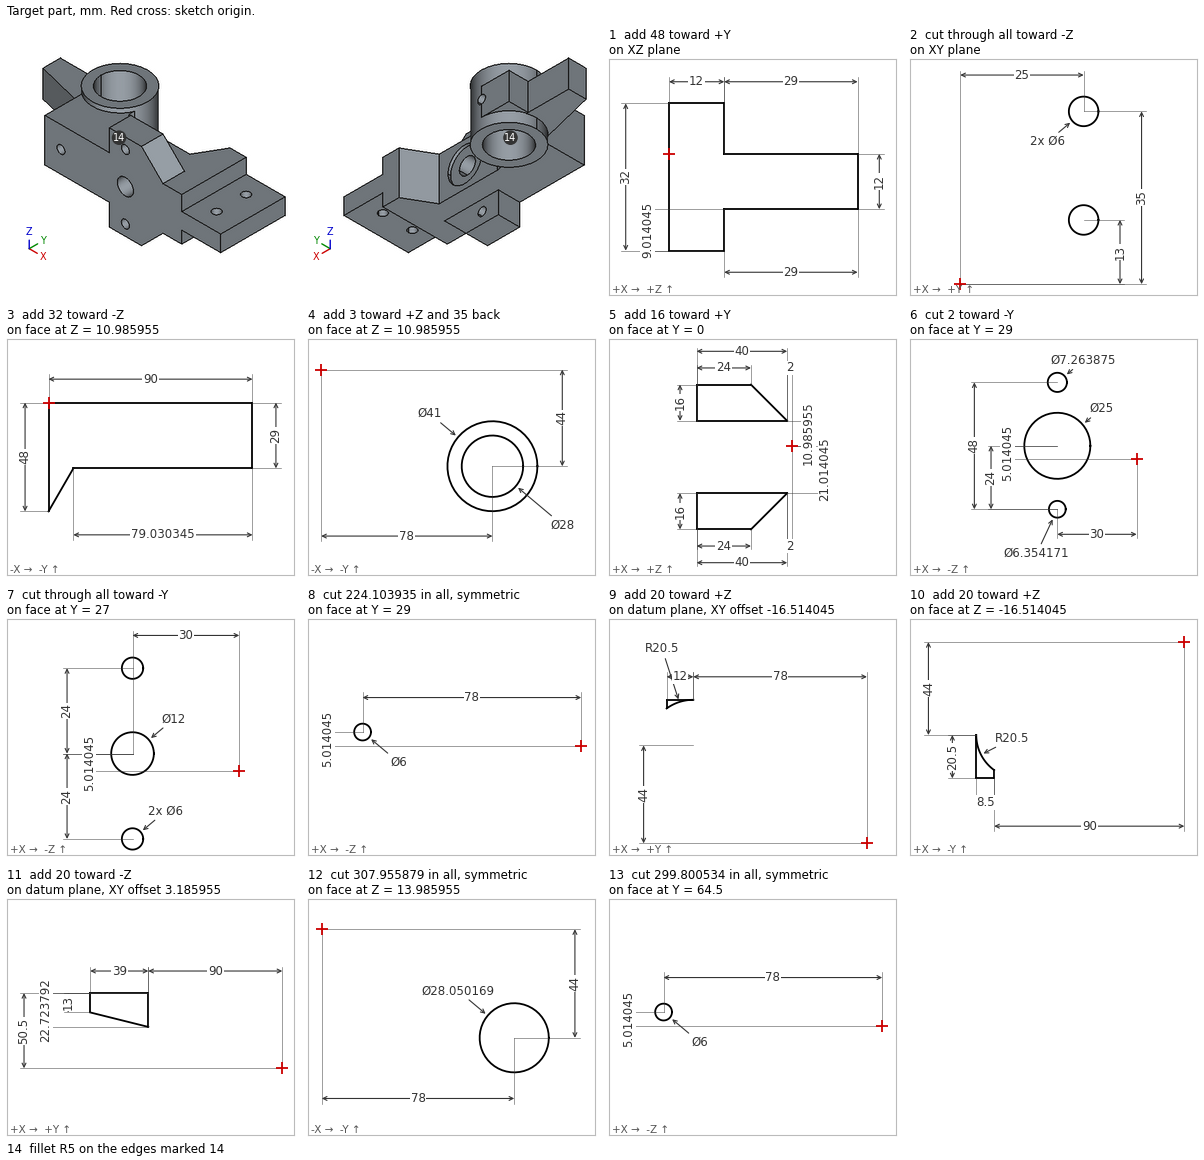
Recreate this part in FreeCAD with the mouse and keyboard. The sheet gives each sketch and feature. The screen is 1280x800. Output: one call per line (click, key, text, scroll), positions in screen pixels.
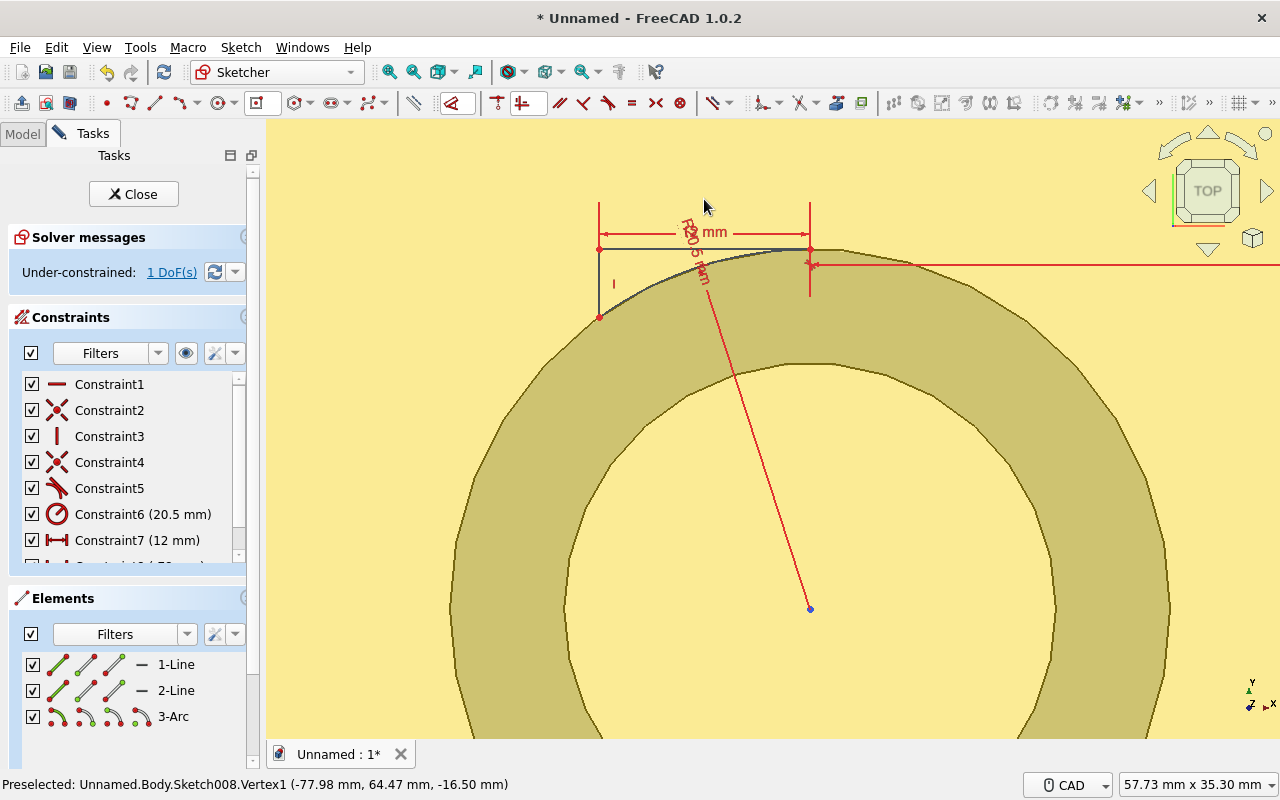
click(810, 609)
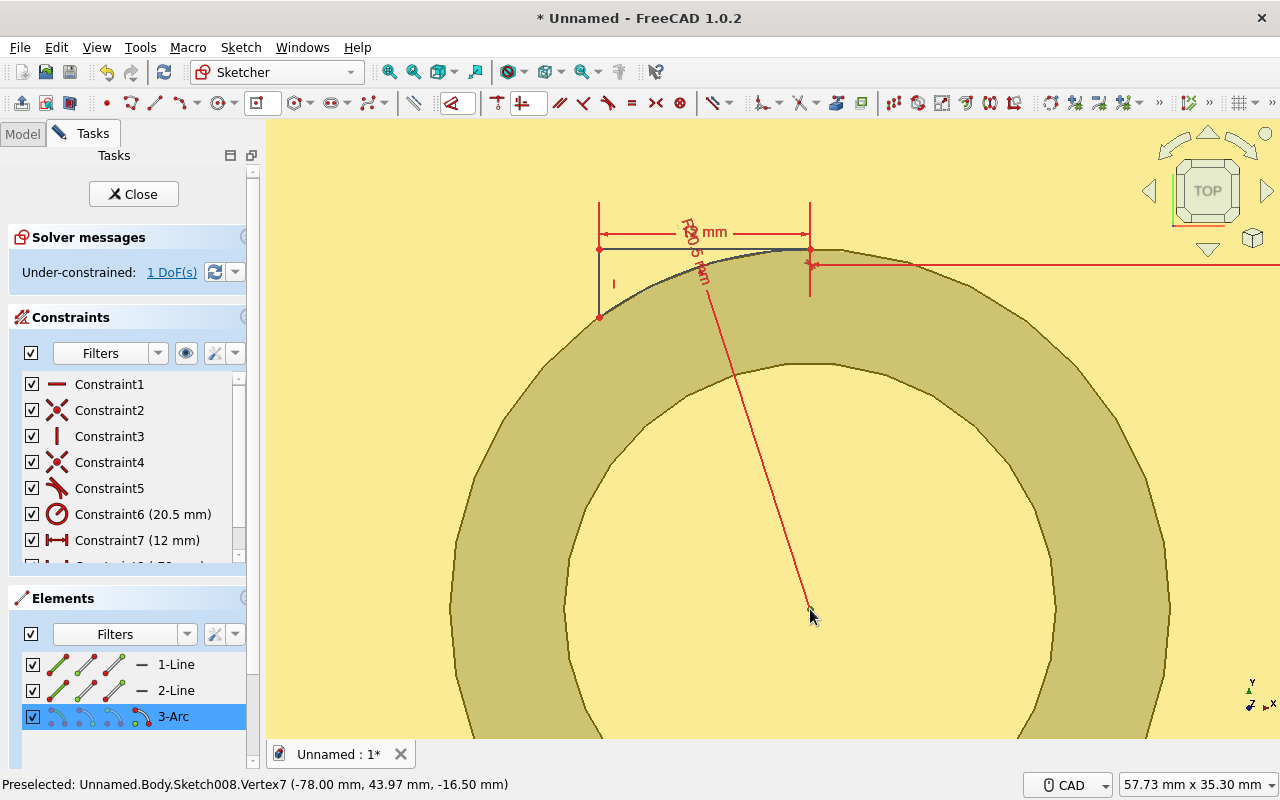
key(i)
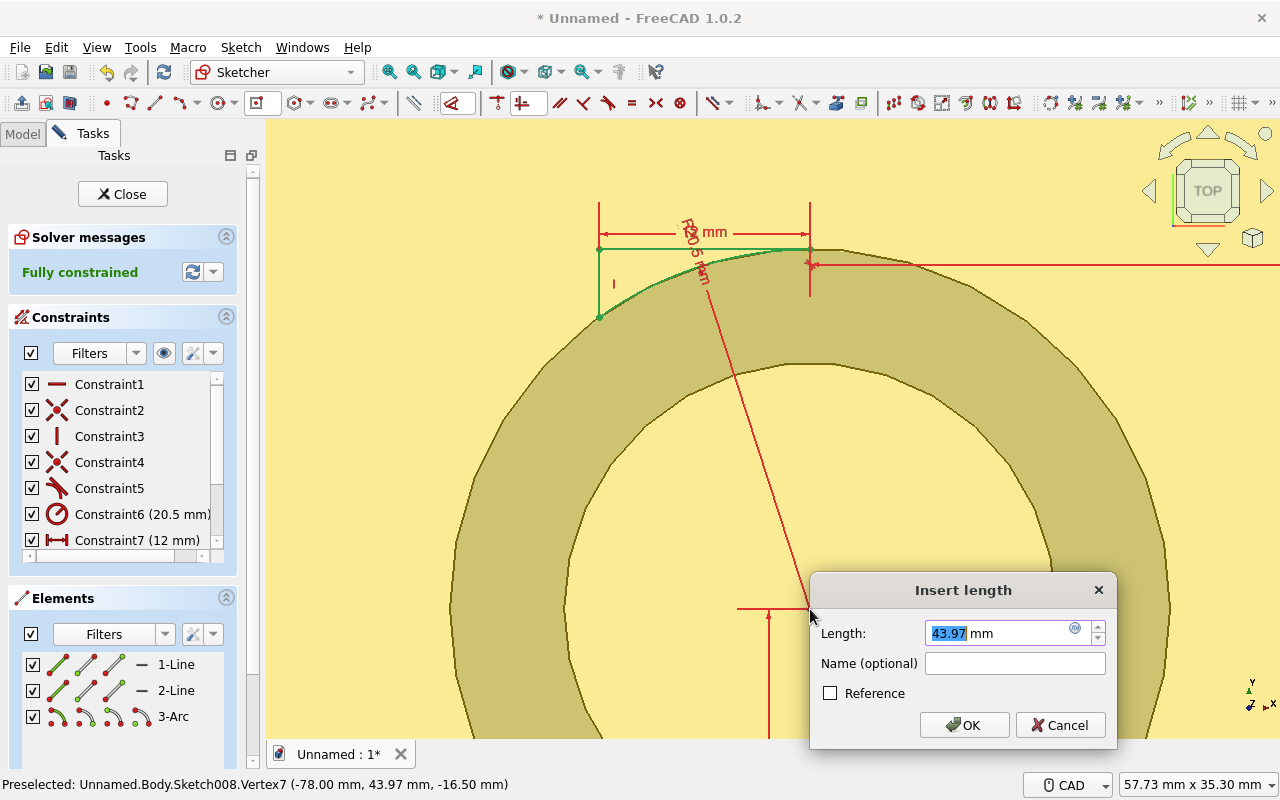
text(44)
key(Return)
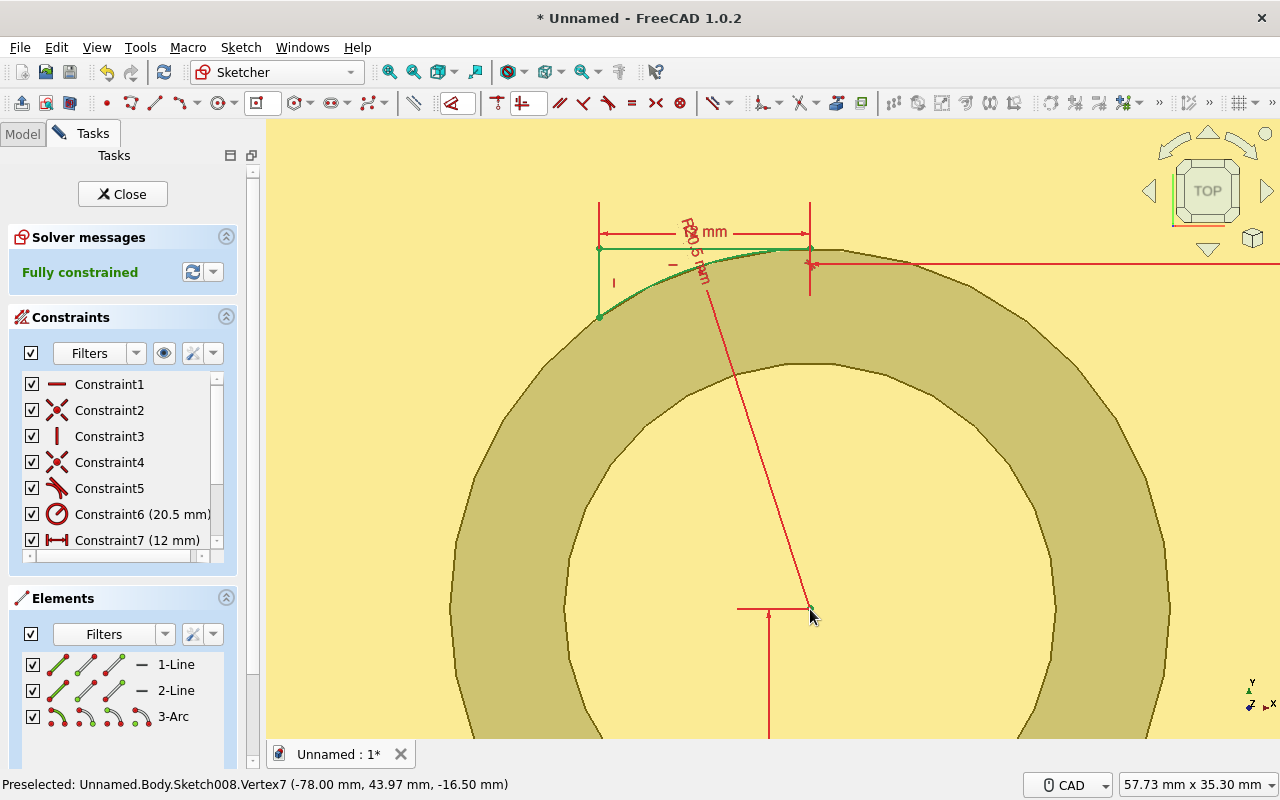
click(123, 194)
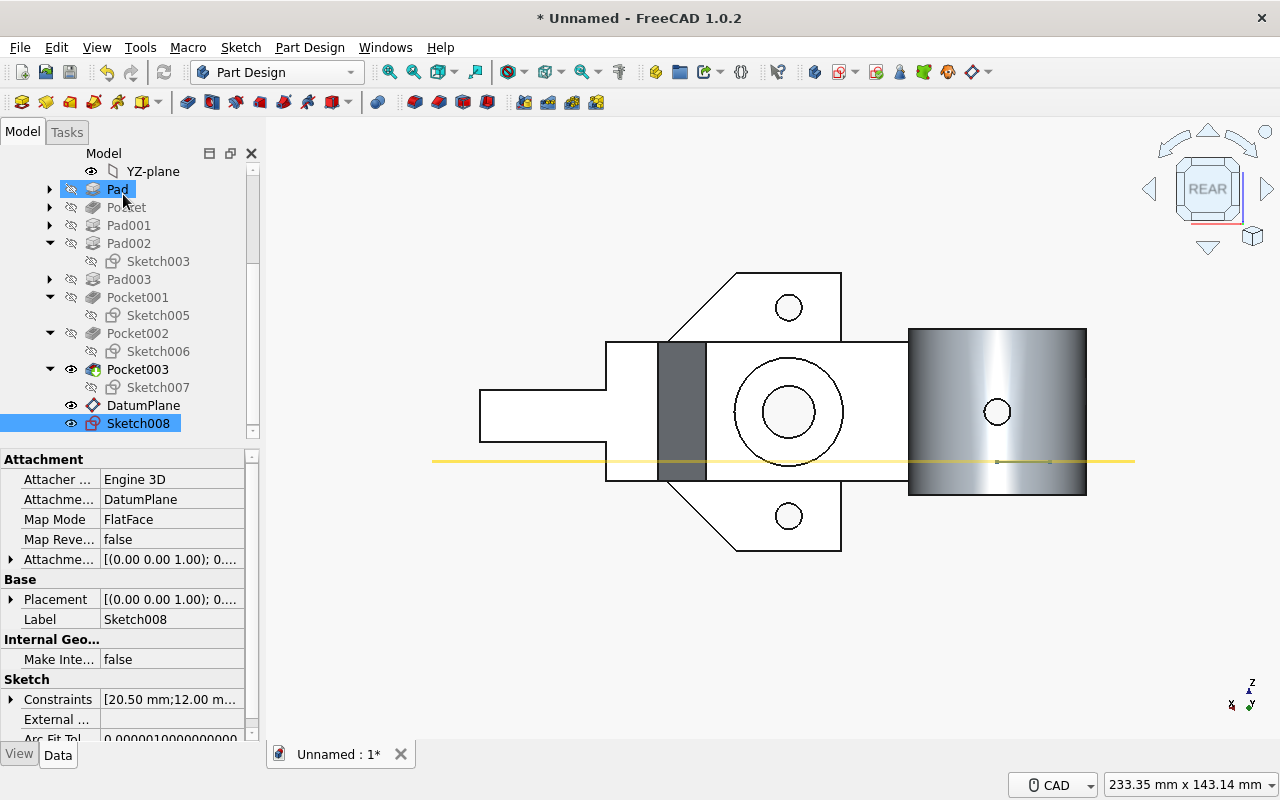
click(22, 102)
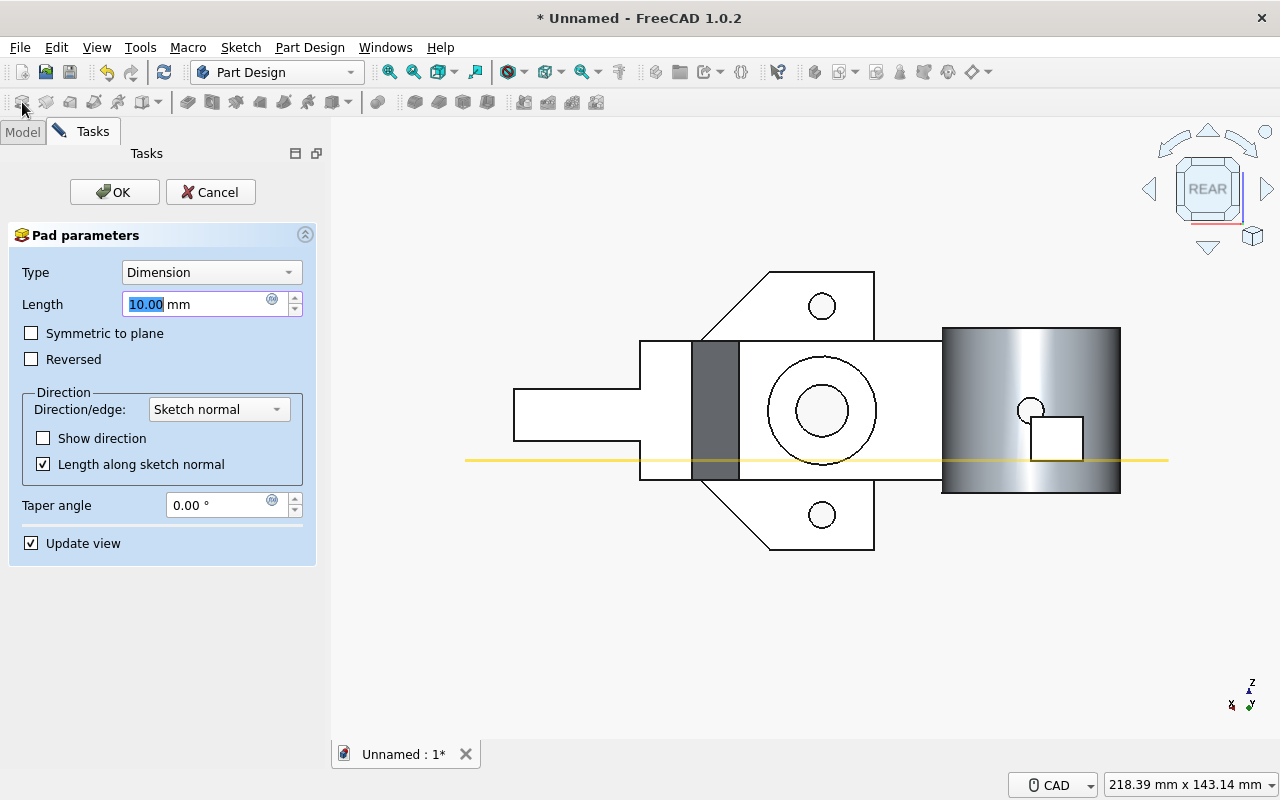
text(20)
key(Tab)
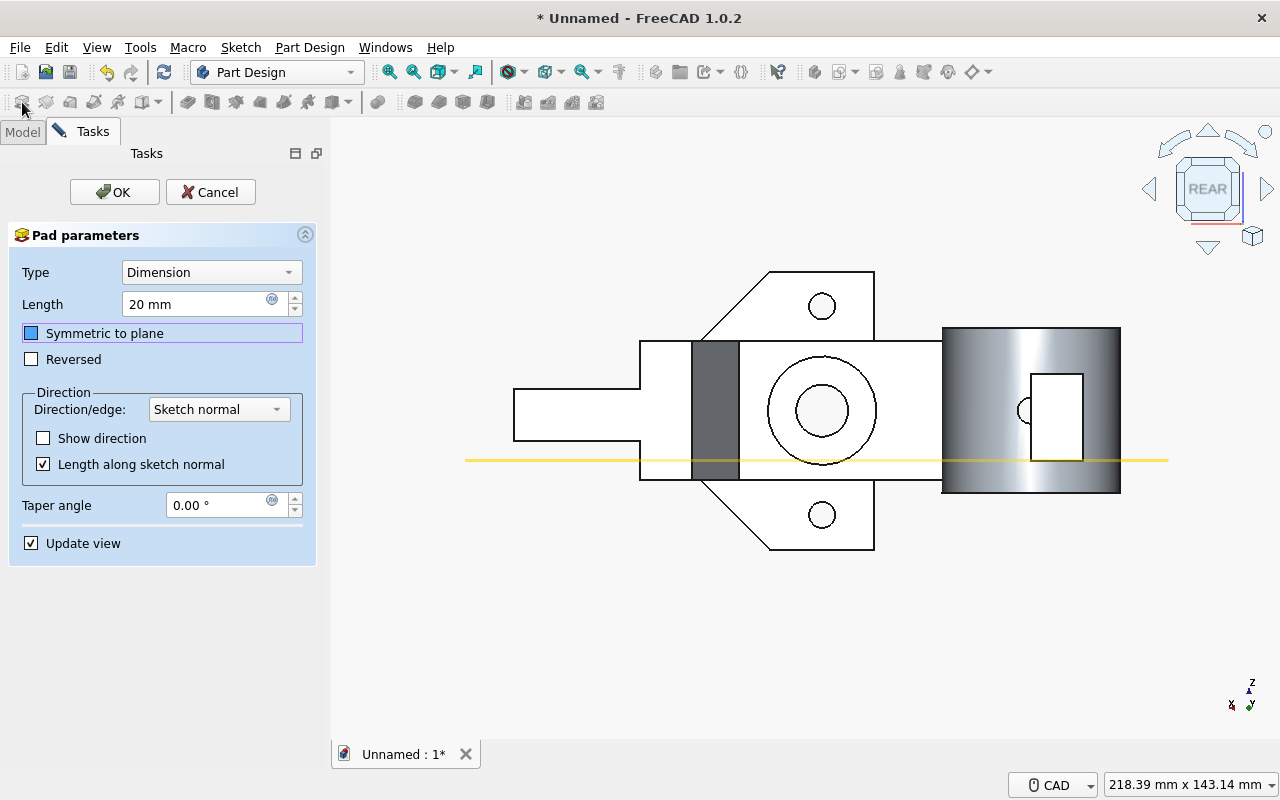
click(115, 192)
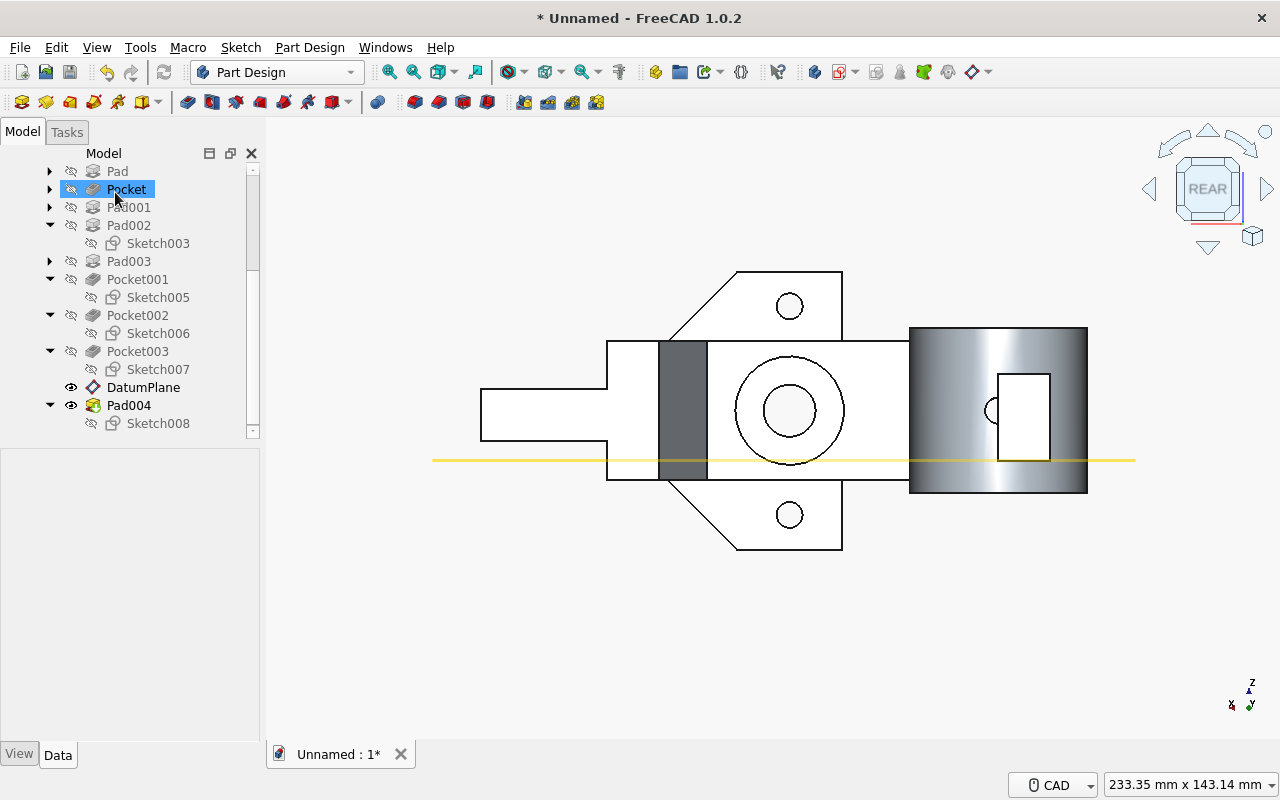
click(116, 387)
key(space)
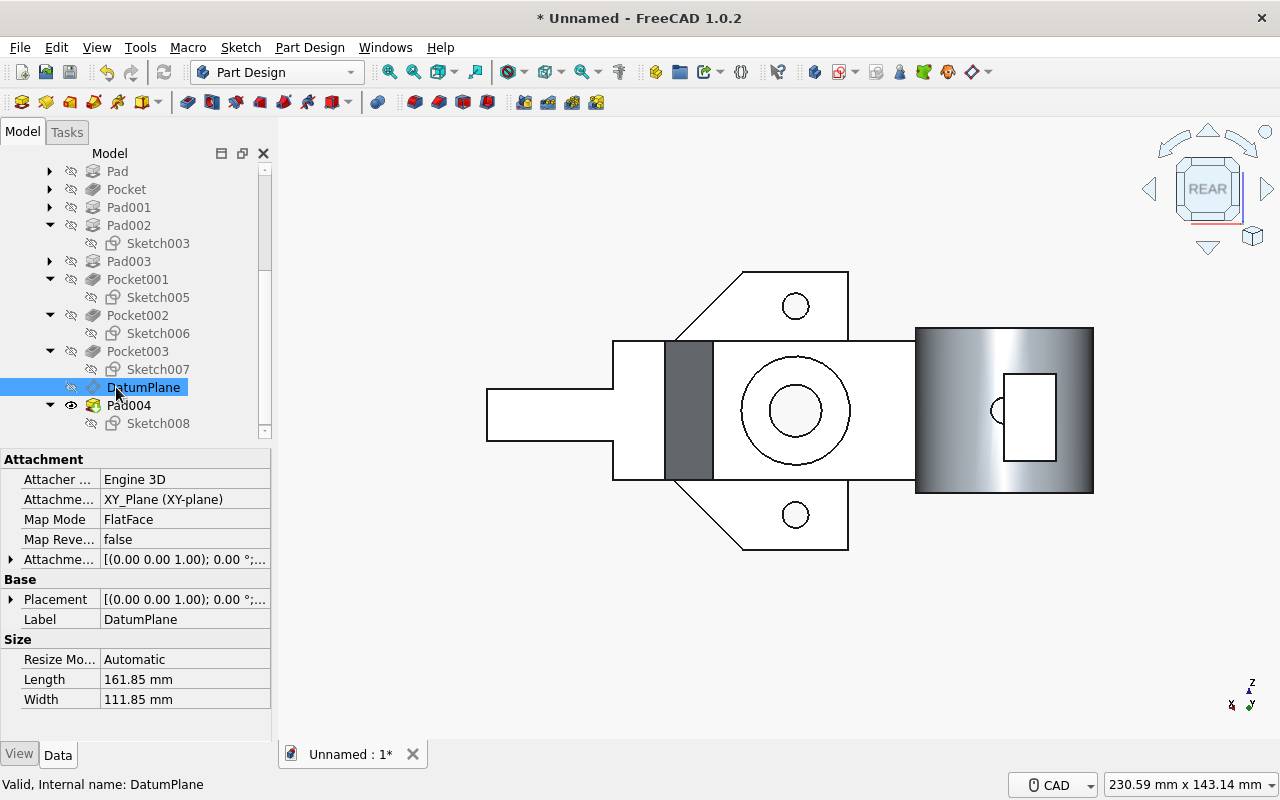
key(5)